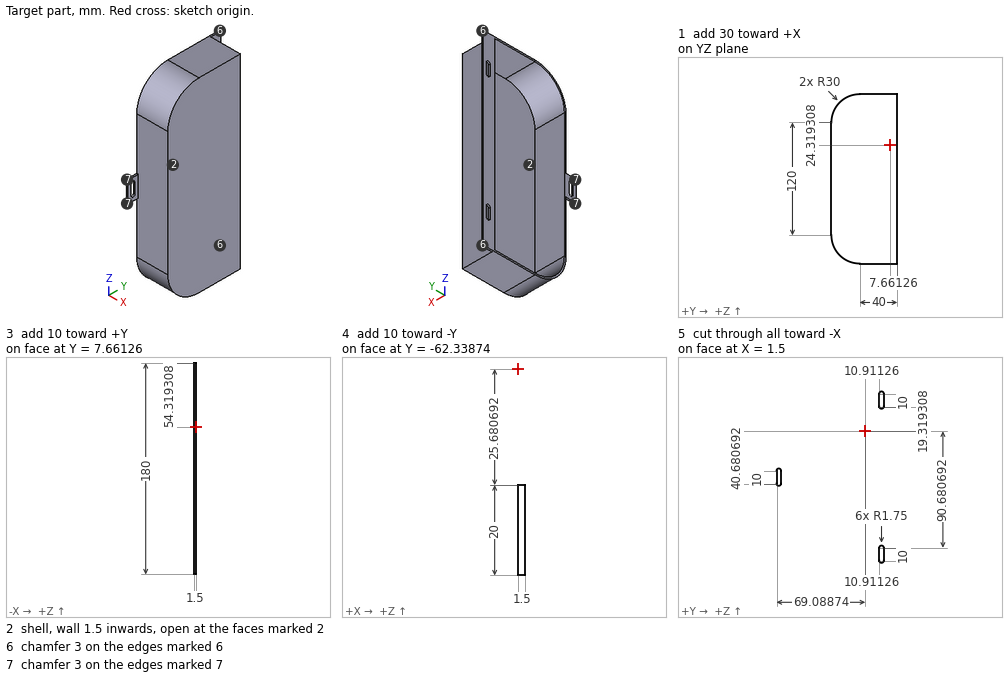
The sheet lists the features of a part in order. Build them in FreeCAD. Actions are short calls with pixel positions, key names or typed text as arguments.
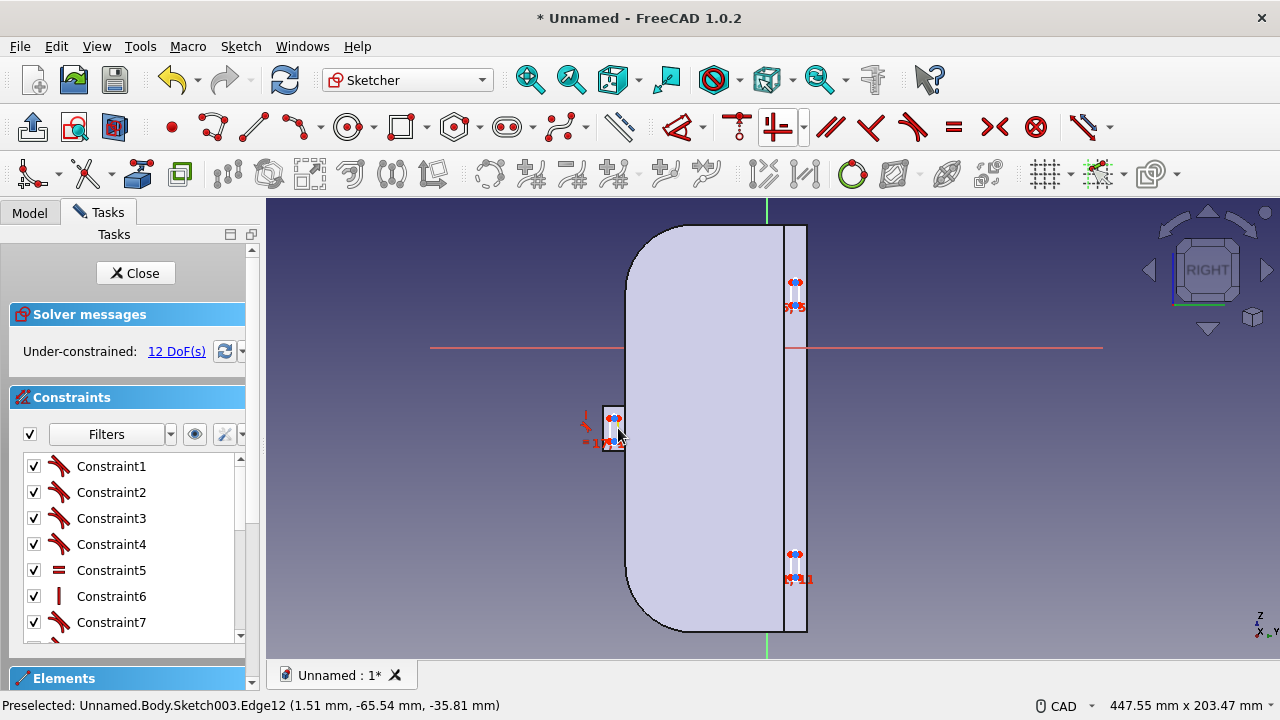
scroll(793, 308, up, 7)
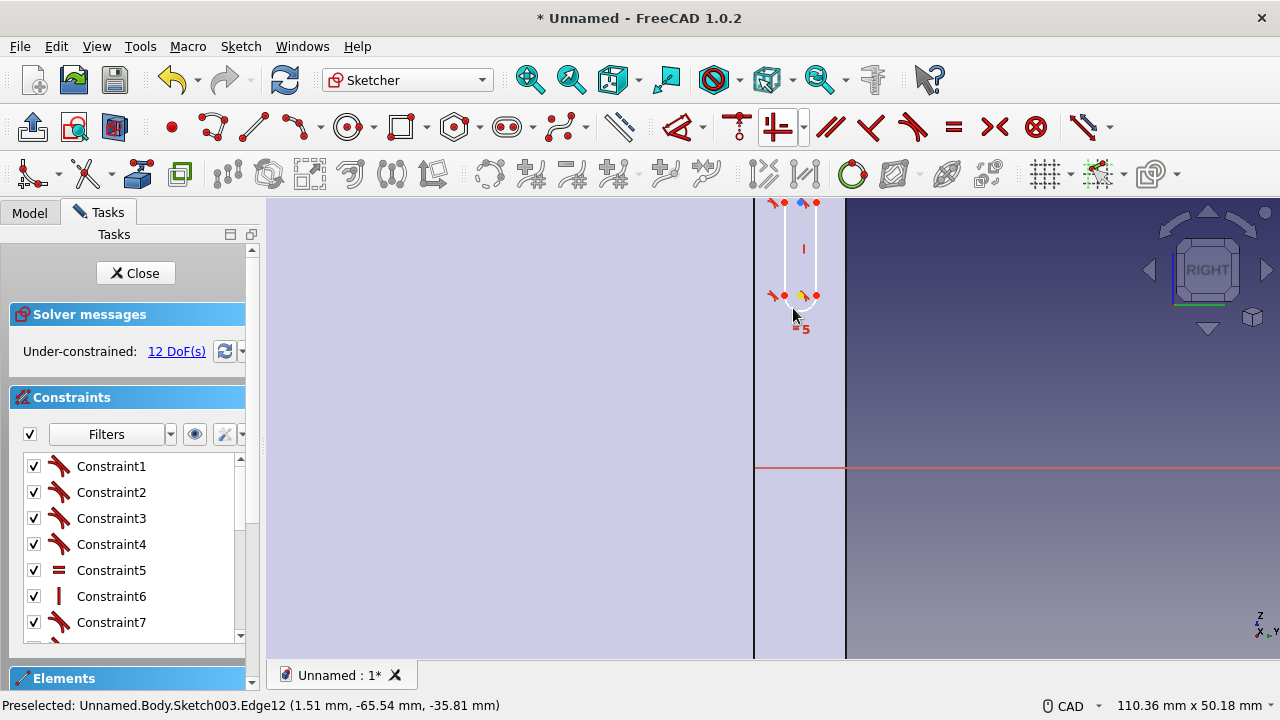
click(791, 308)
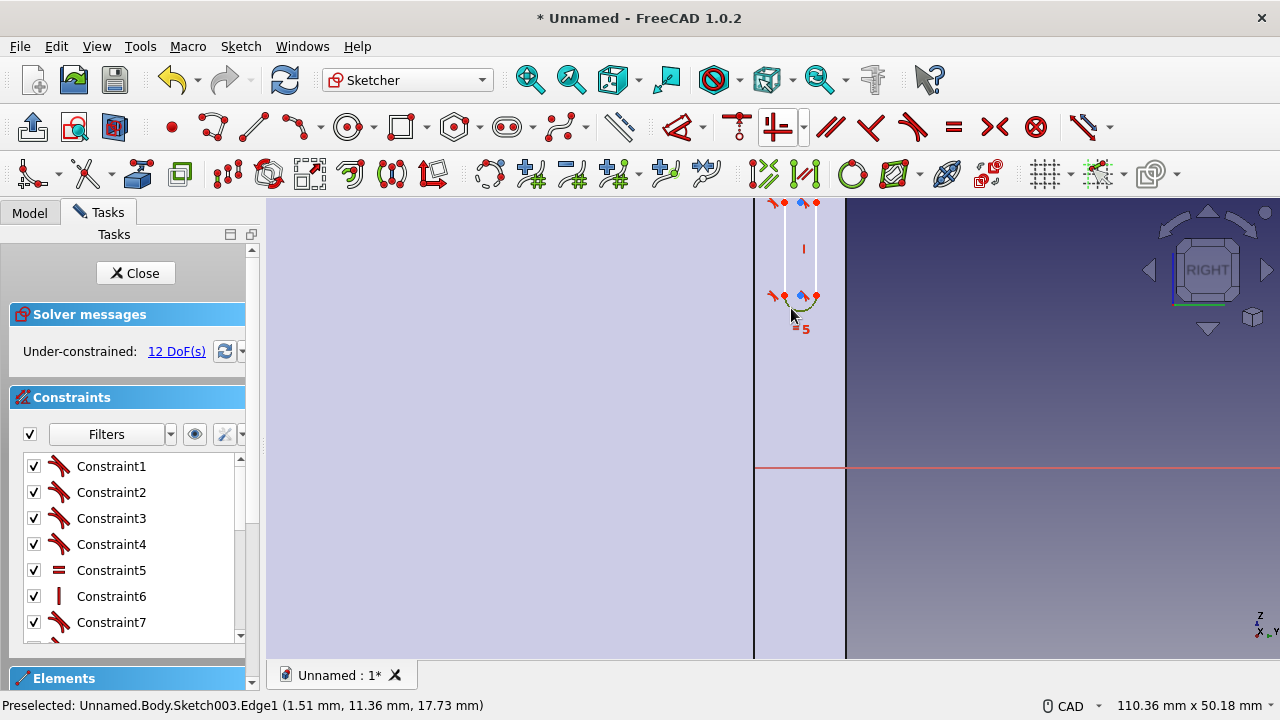
scroll(793, 308, down, 7)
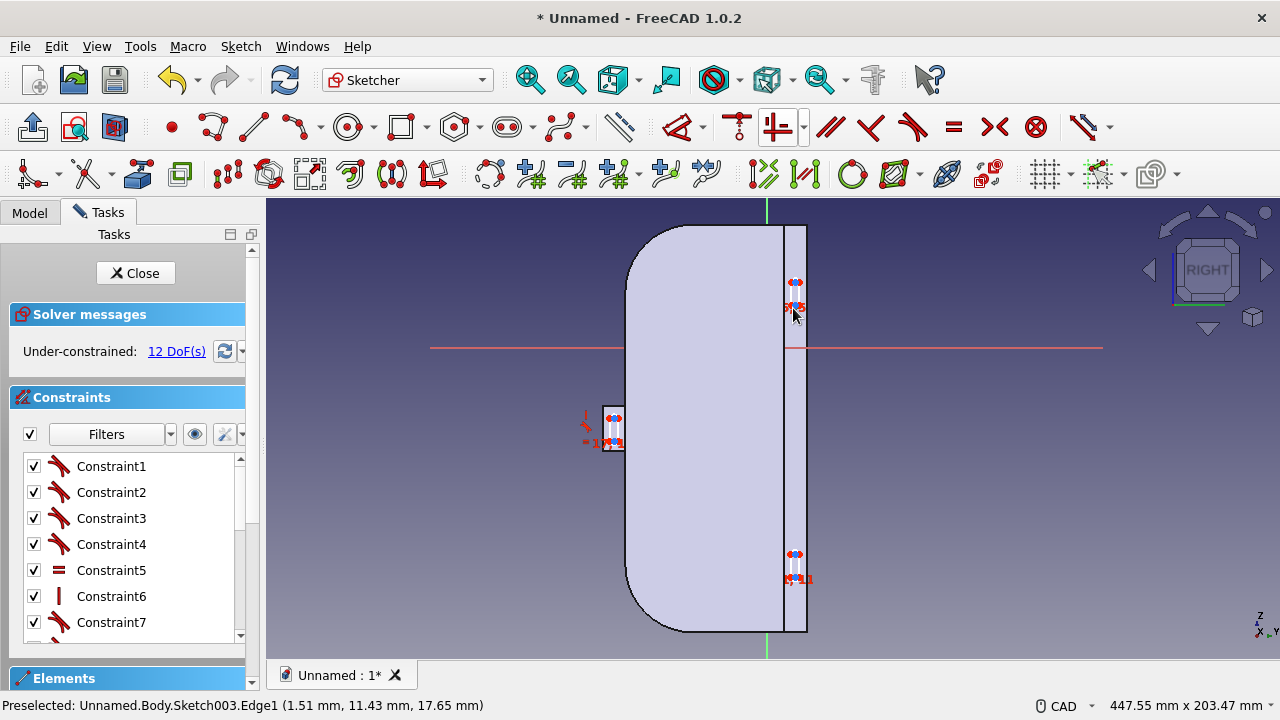
scroll(793, 581, up, 7)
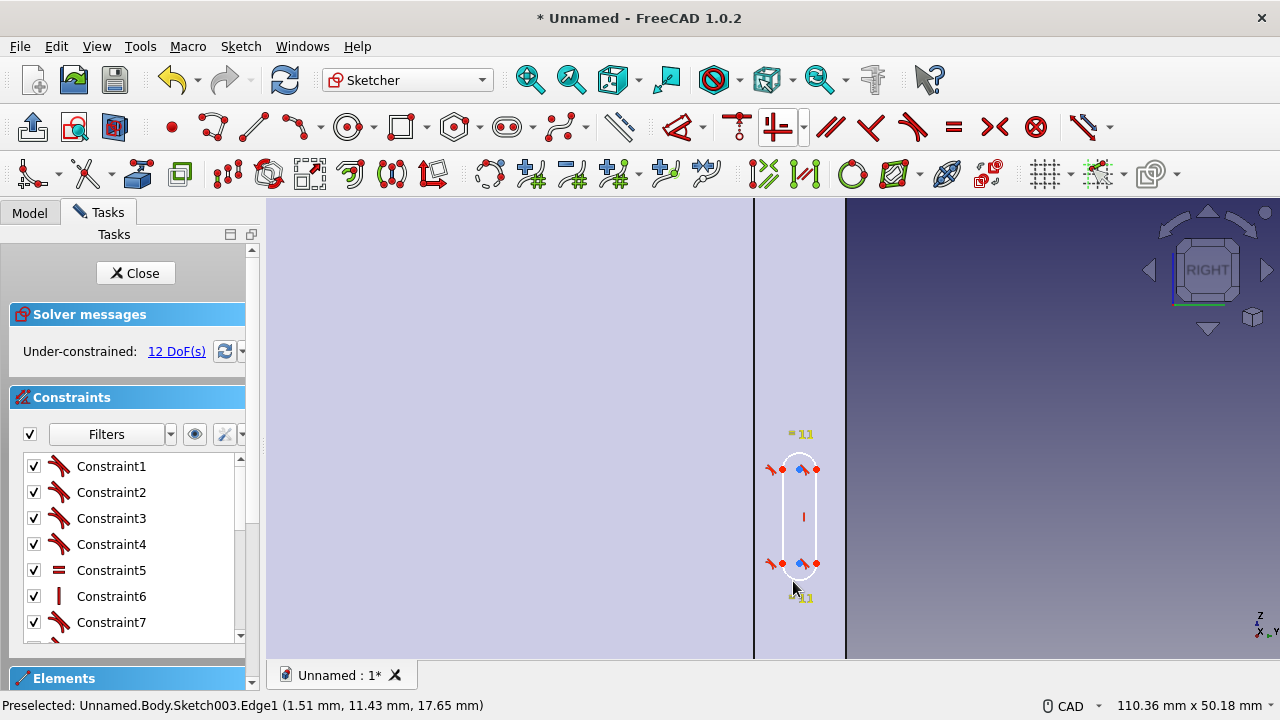
click(790, 577)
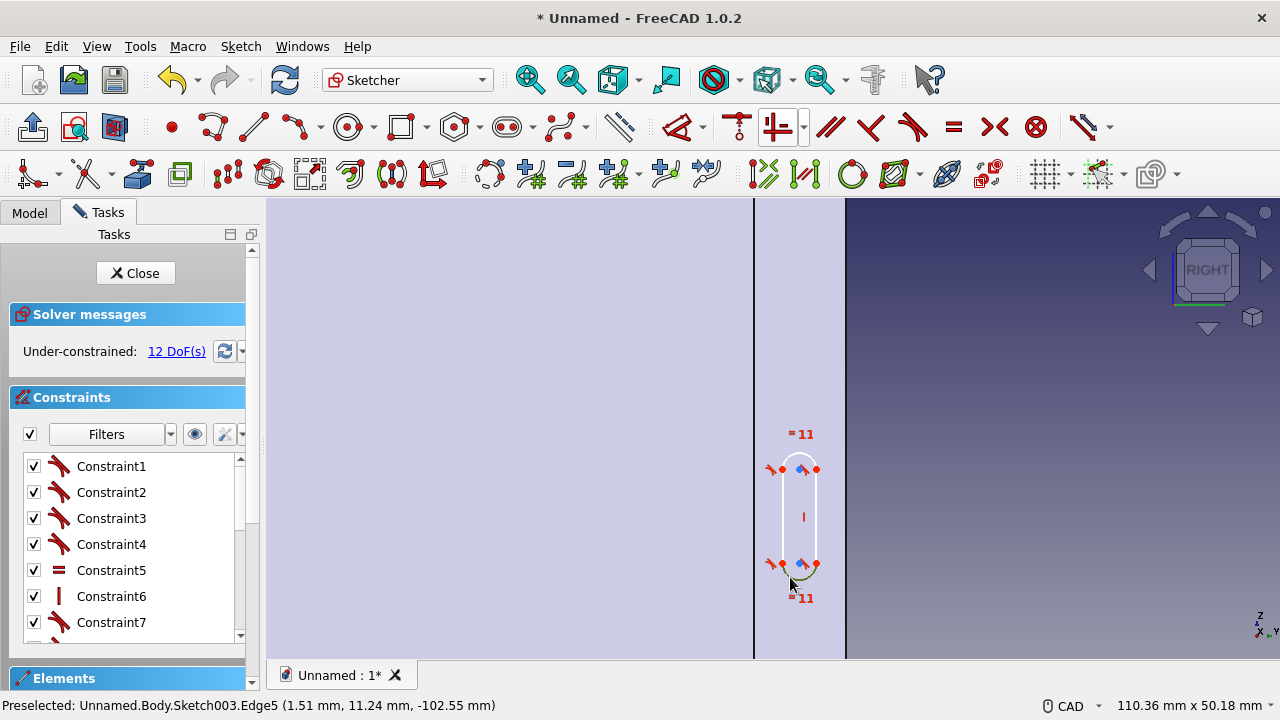
scroll(793, 582, down, 7)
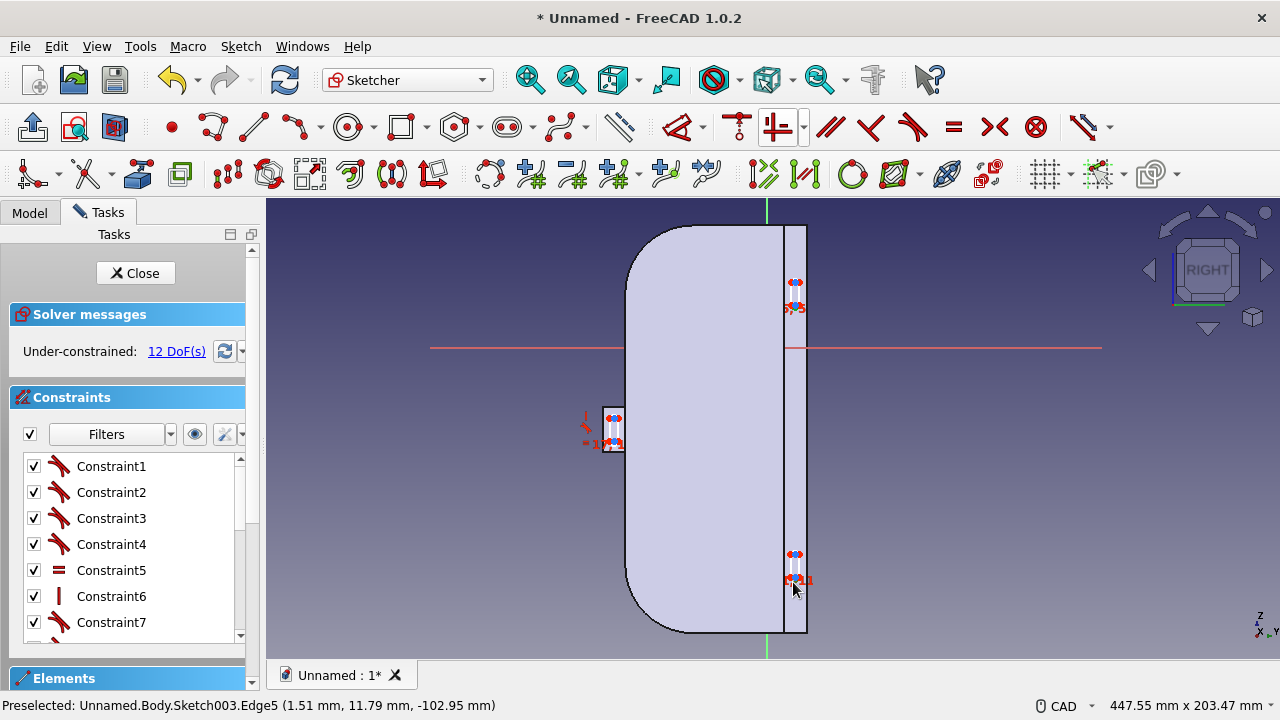
scroll(612, 445, up, 7)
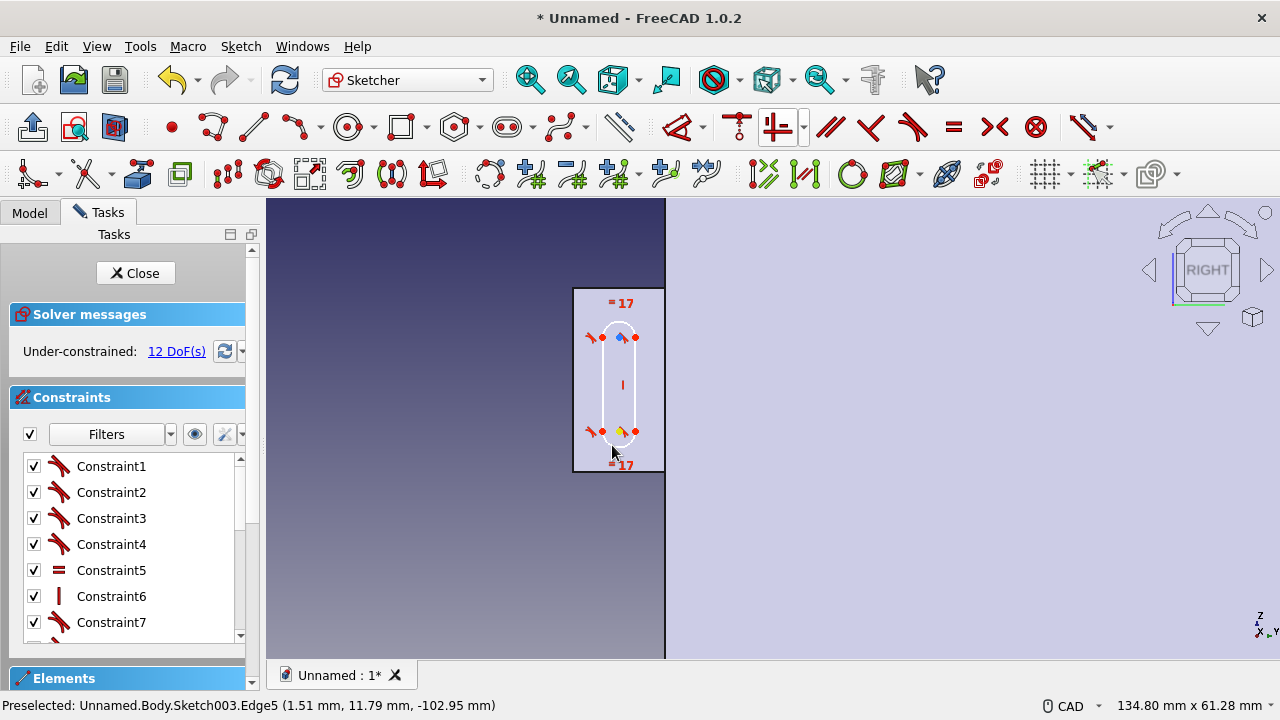
click(609, 444)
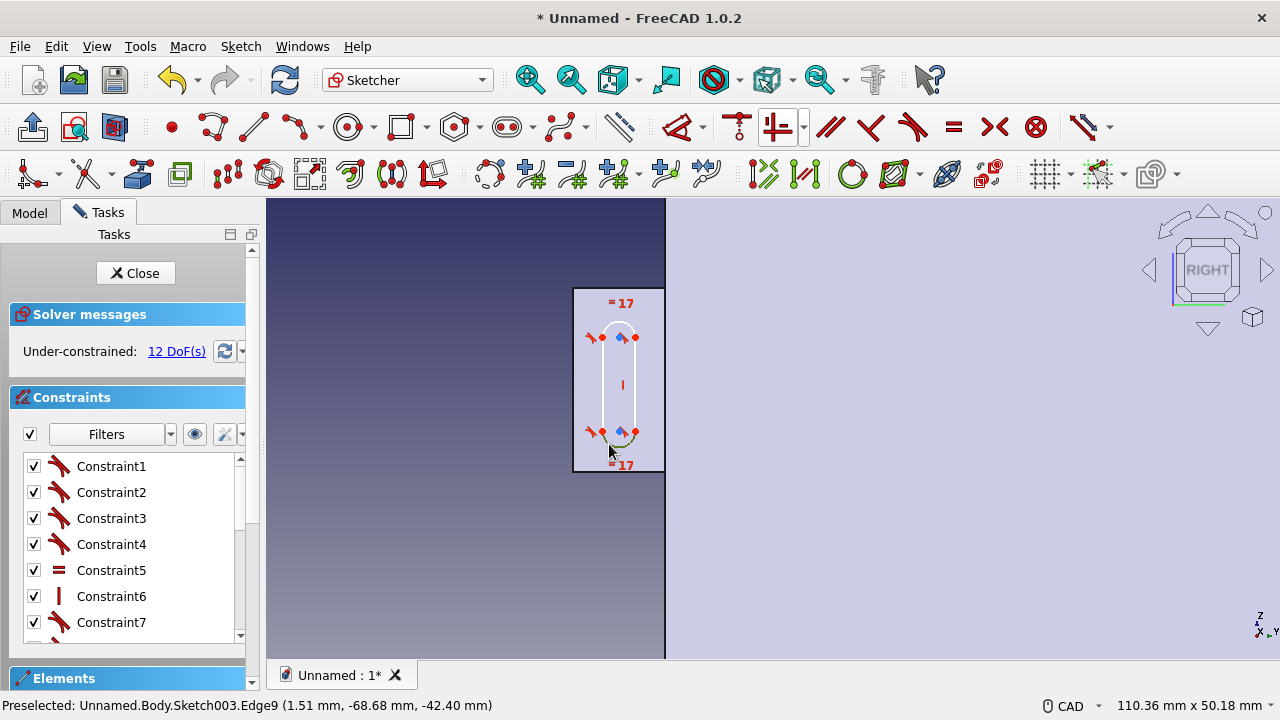
click(954, 128)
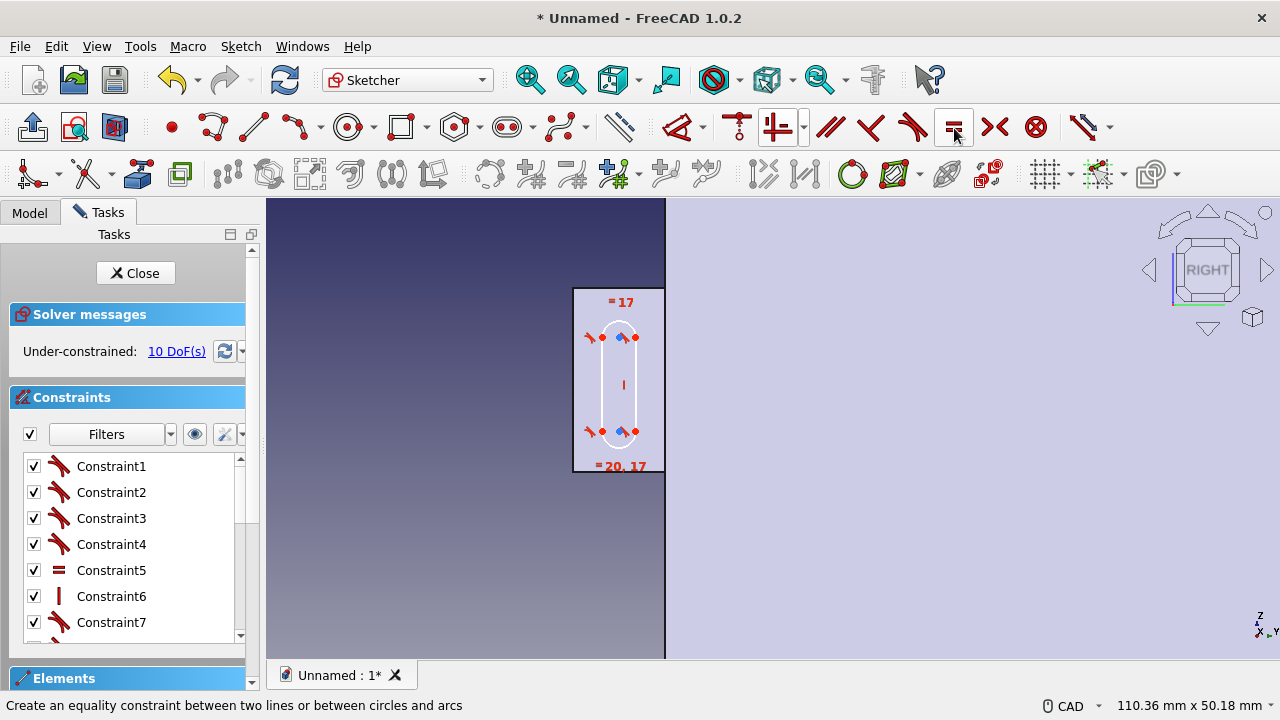
click(676, 128)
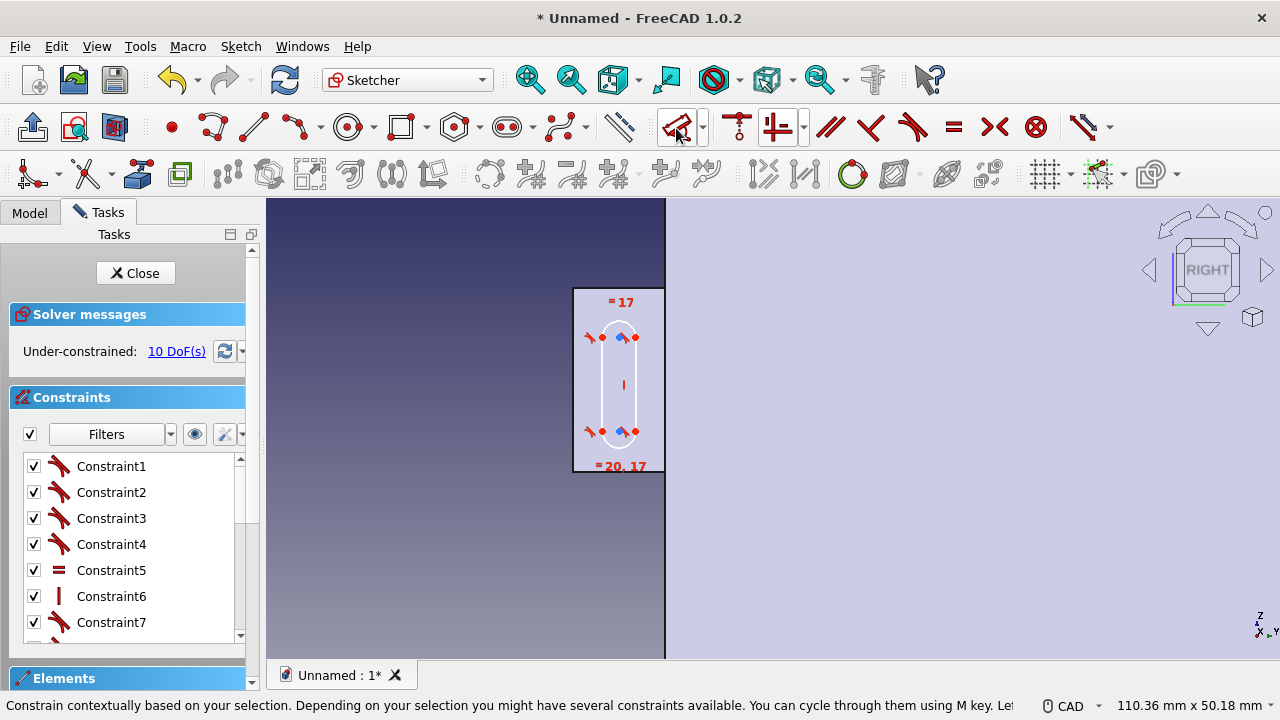
scroll(612, 444, down, 7)